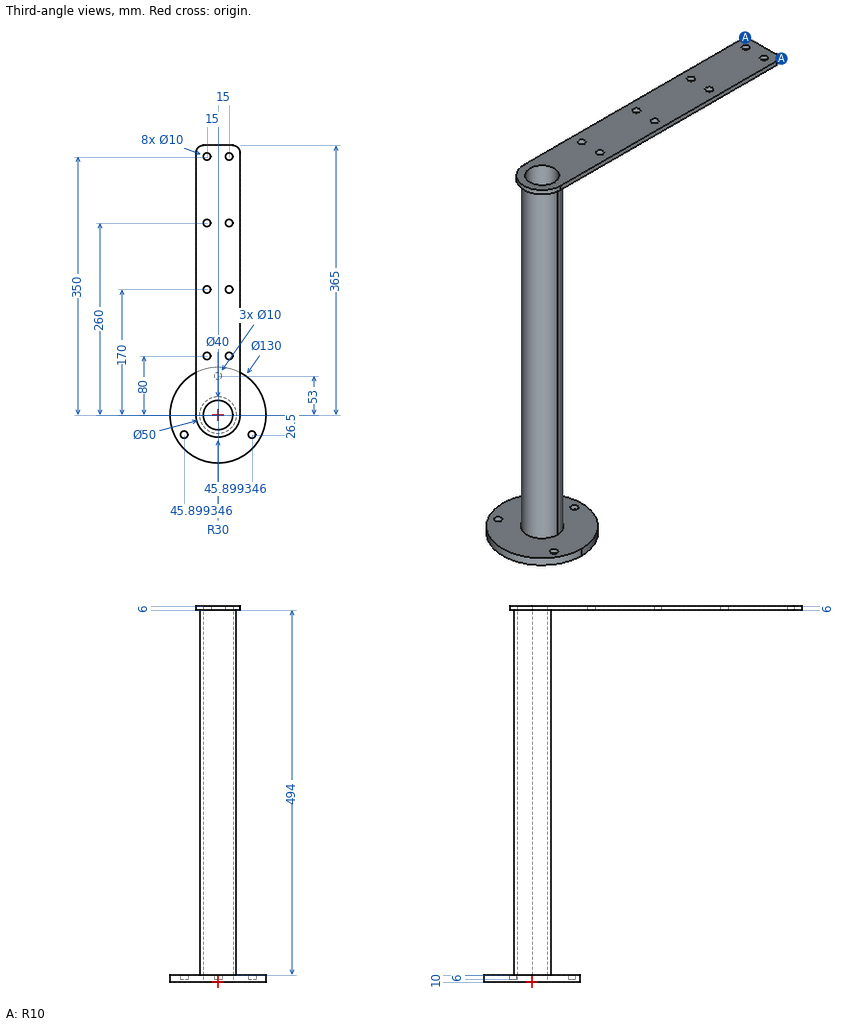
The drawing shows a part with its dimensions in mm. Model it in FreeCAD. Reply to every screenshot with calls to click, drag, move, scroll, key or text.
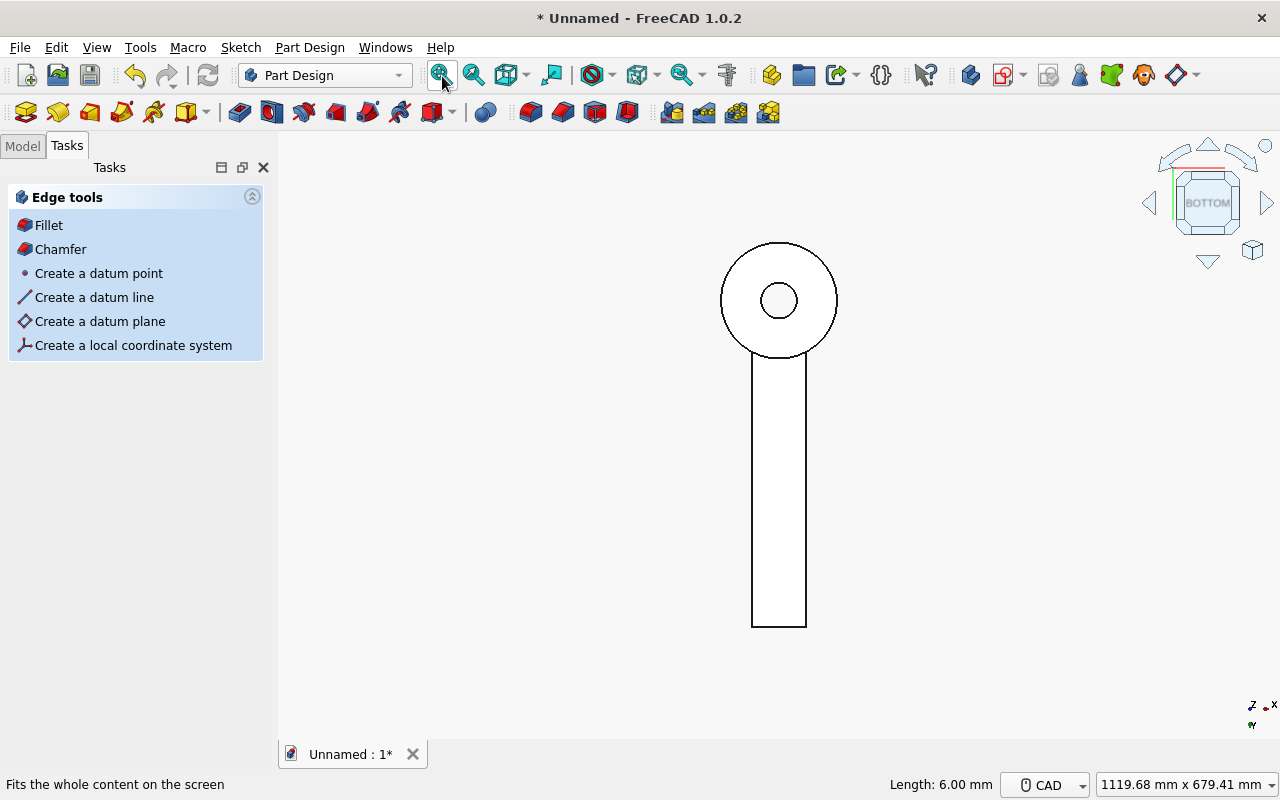
scroll(752, 626, up, 11)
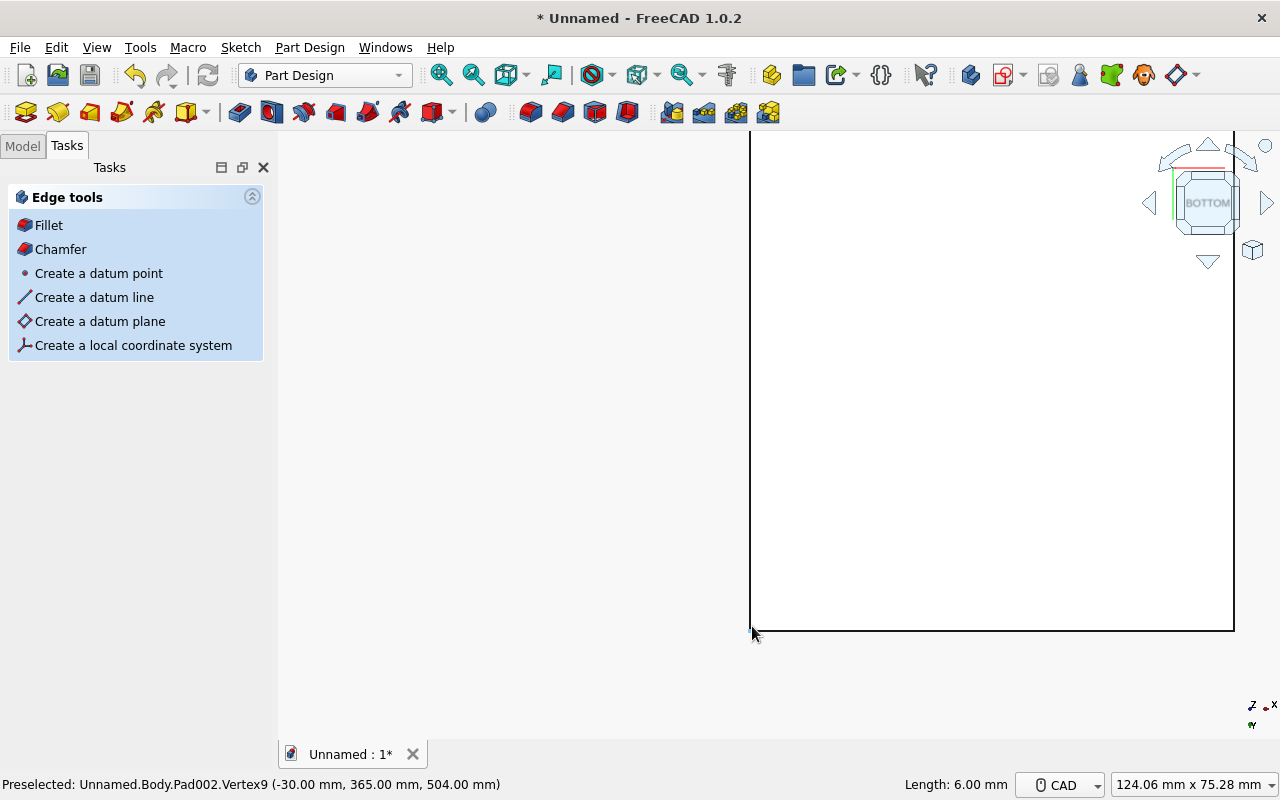
click(442, 76)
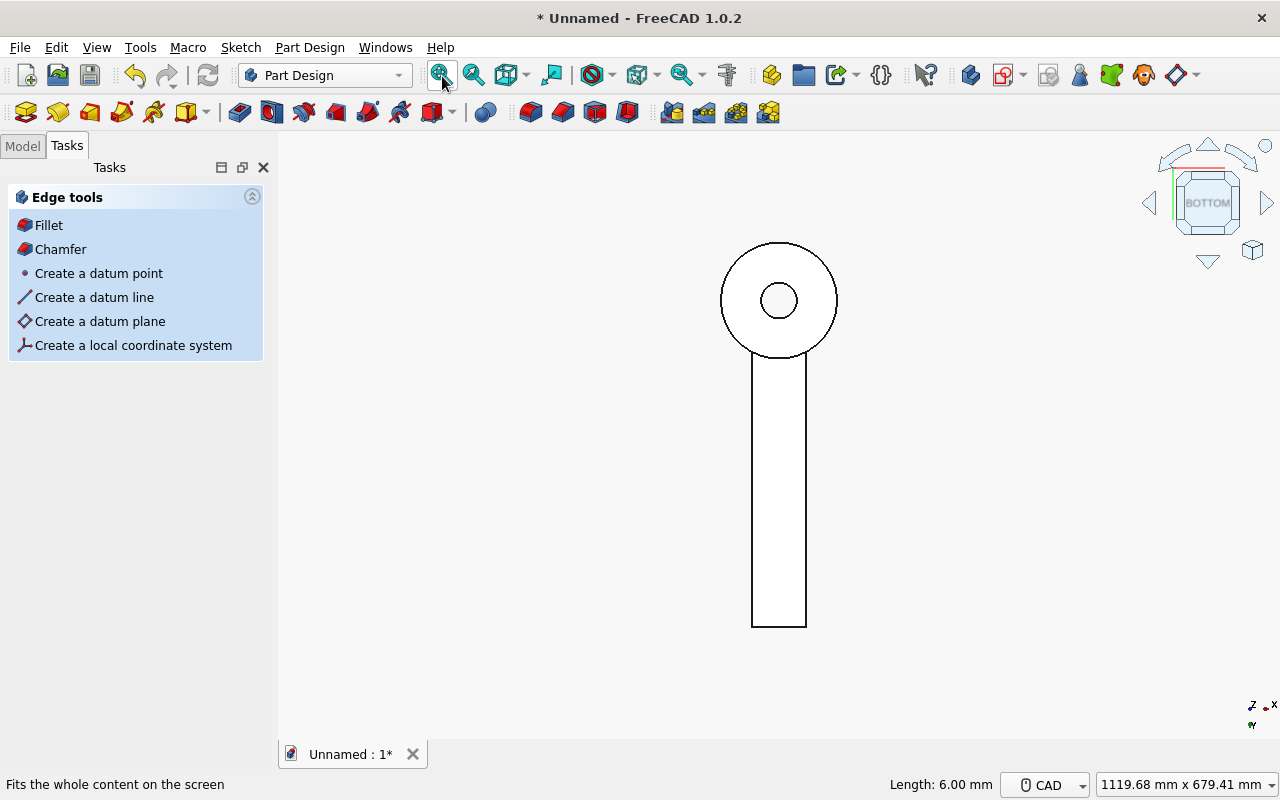
key(4)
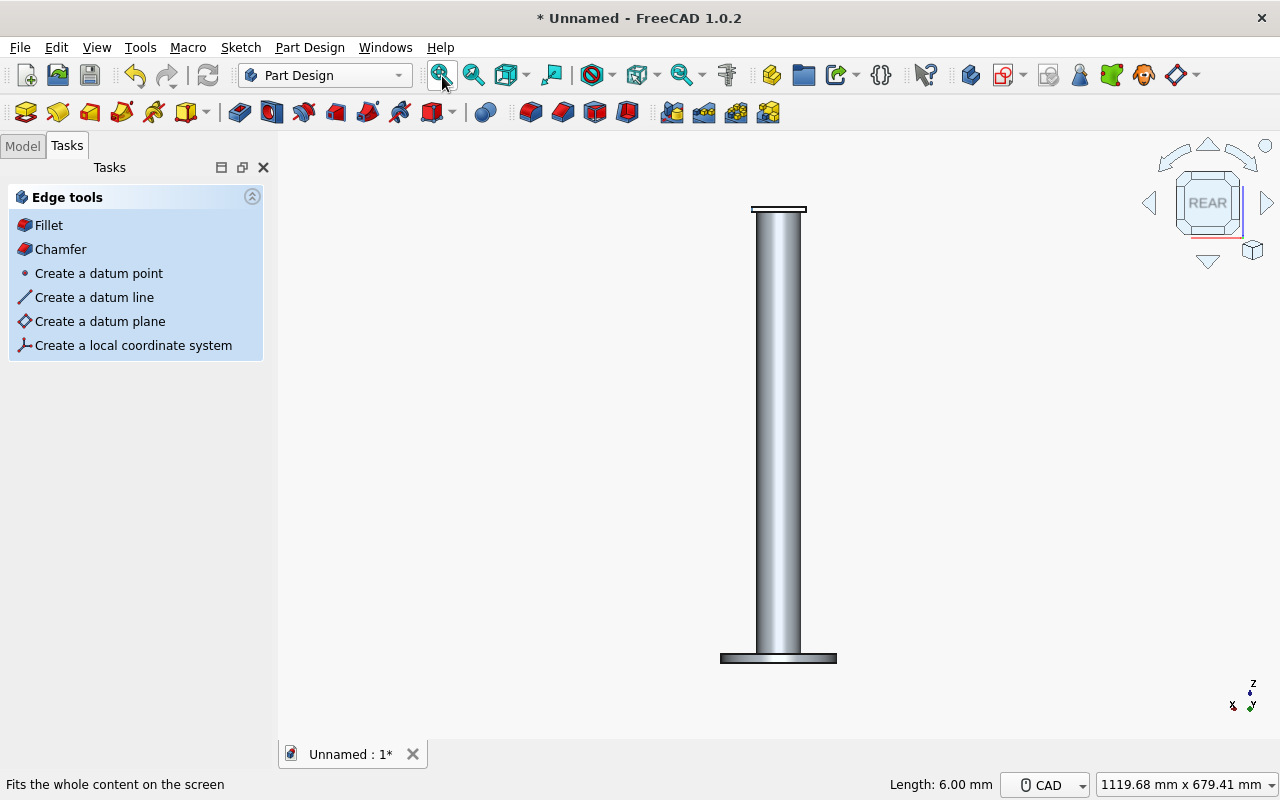
scroll(806, 208, up, 11)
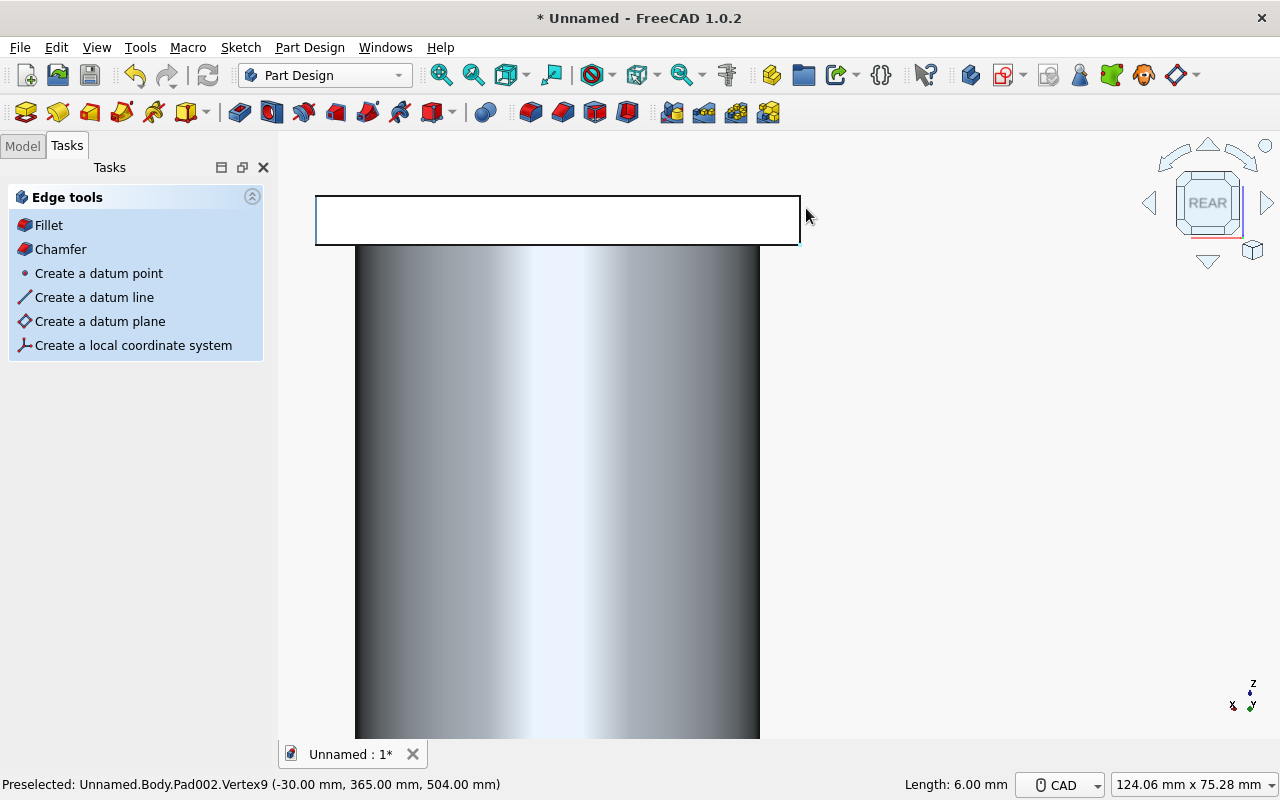
click(800, 219, ctrl)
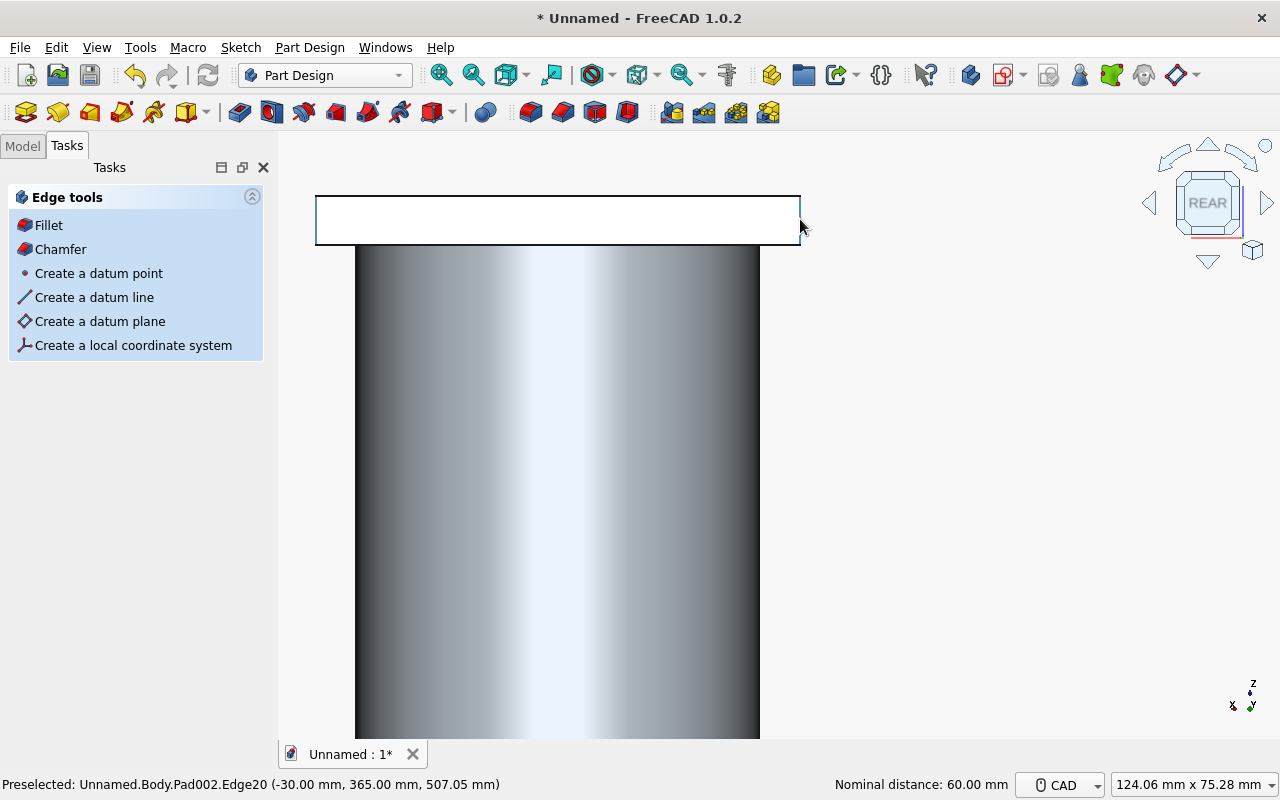
click(532, 112)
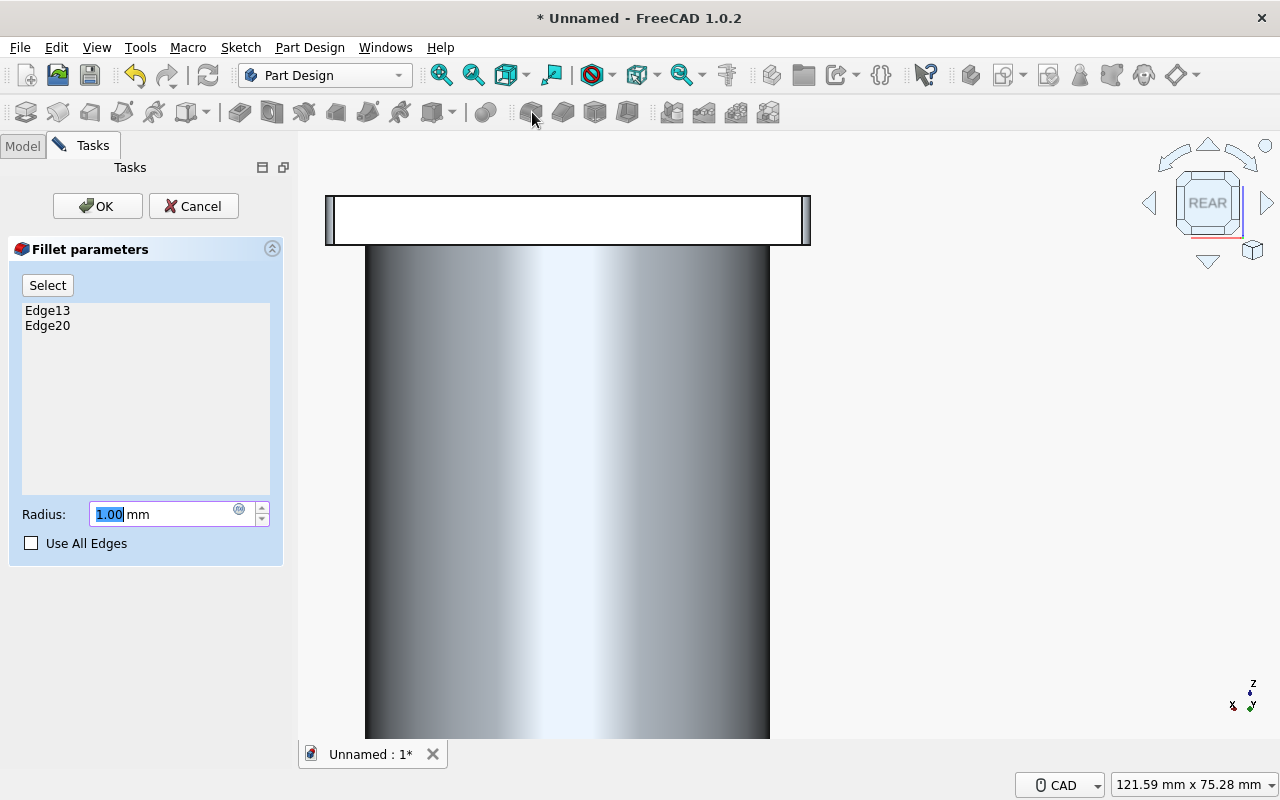
text(10)
key(Tab)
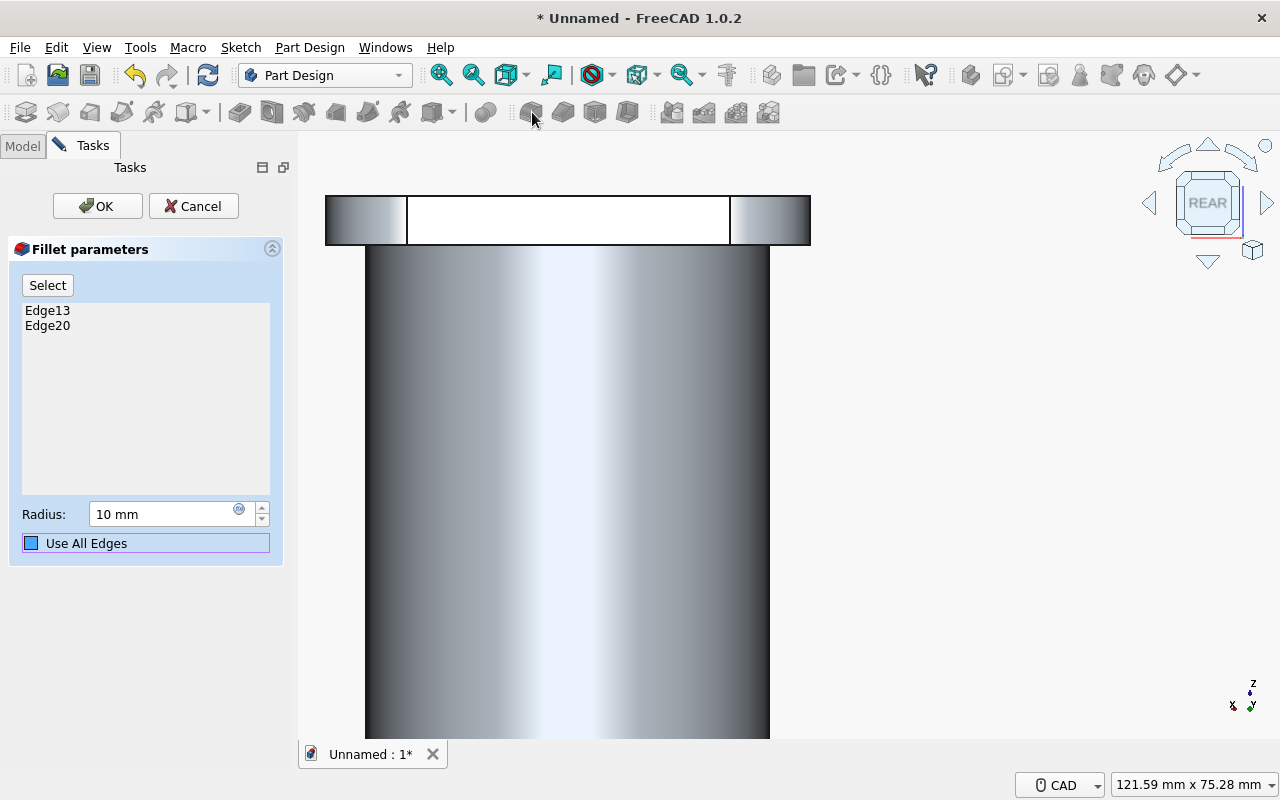
click(98, 206)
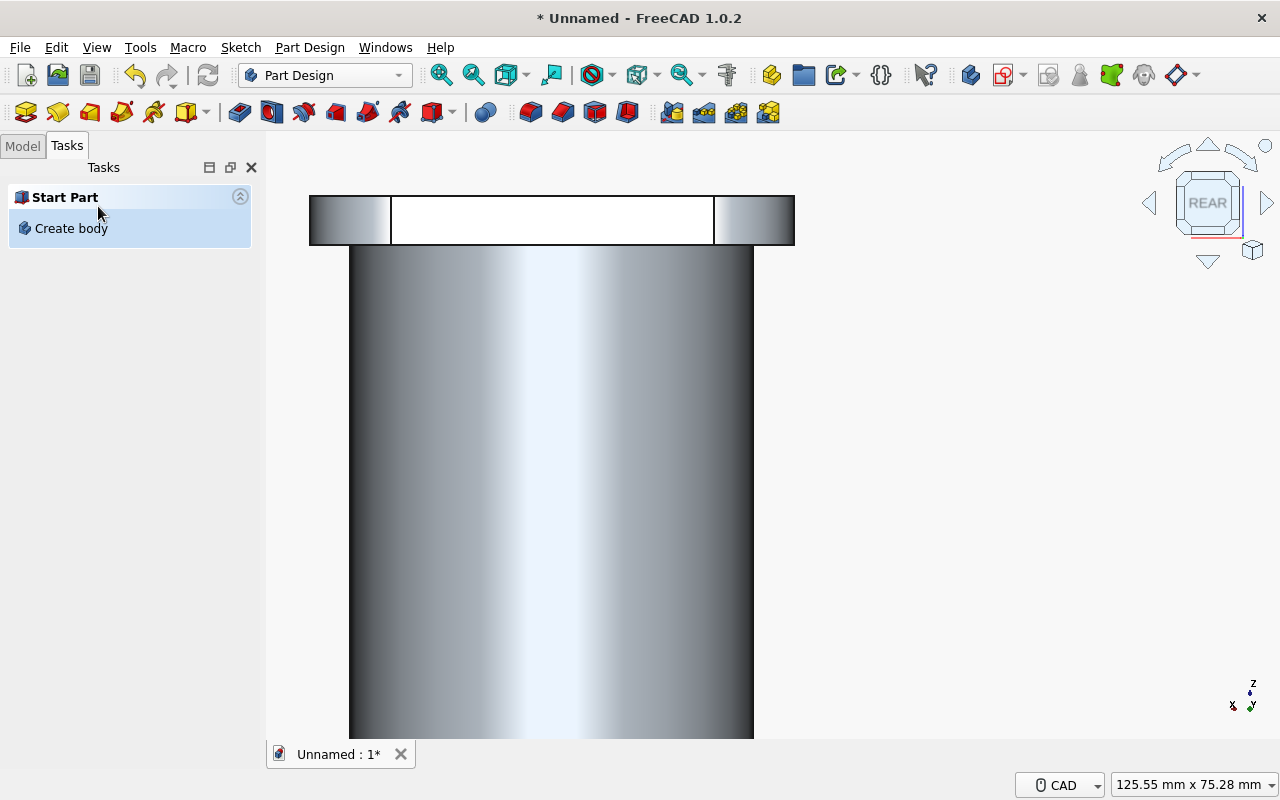
click(442, 76)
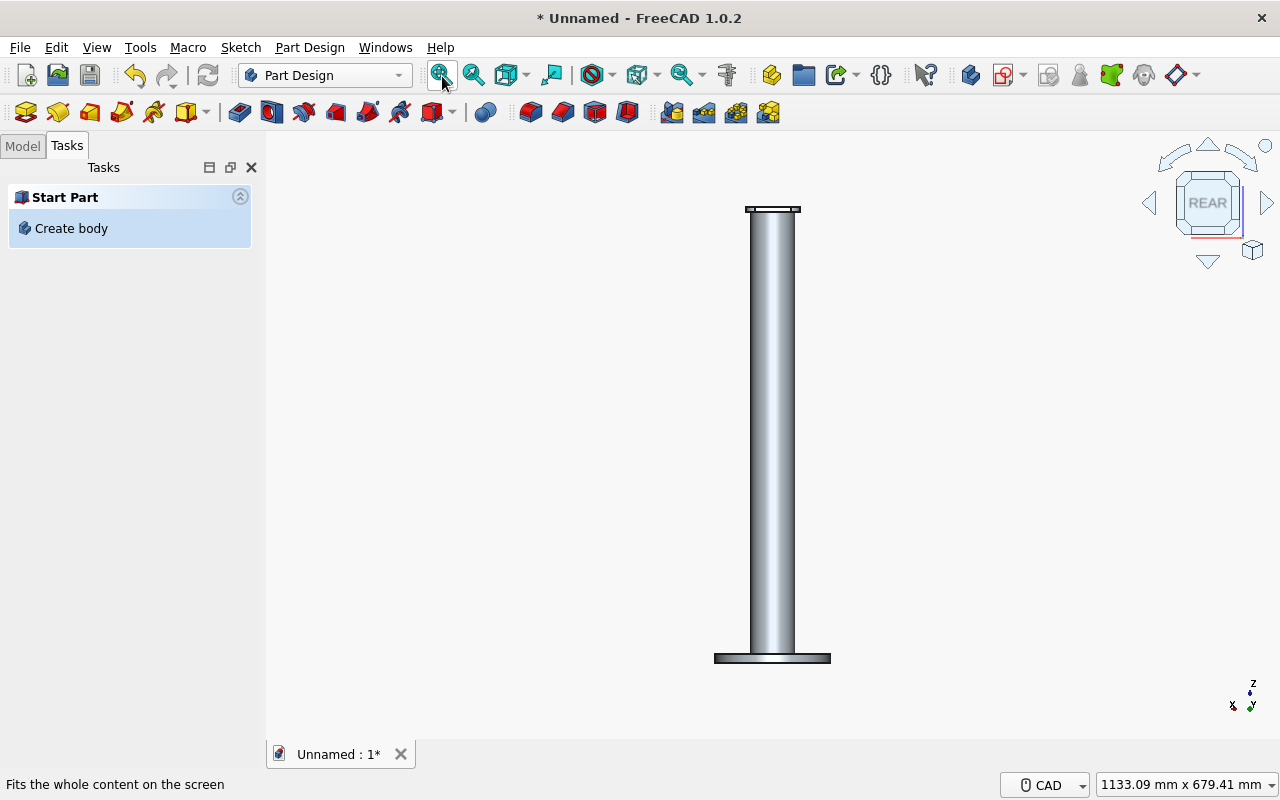
key(0)